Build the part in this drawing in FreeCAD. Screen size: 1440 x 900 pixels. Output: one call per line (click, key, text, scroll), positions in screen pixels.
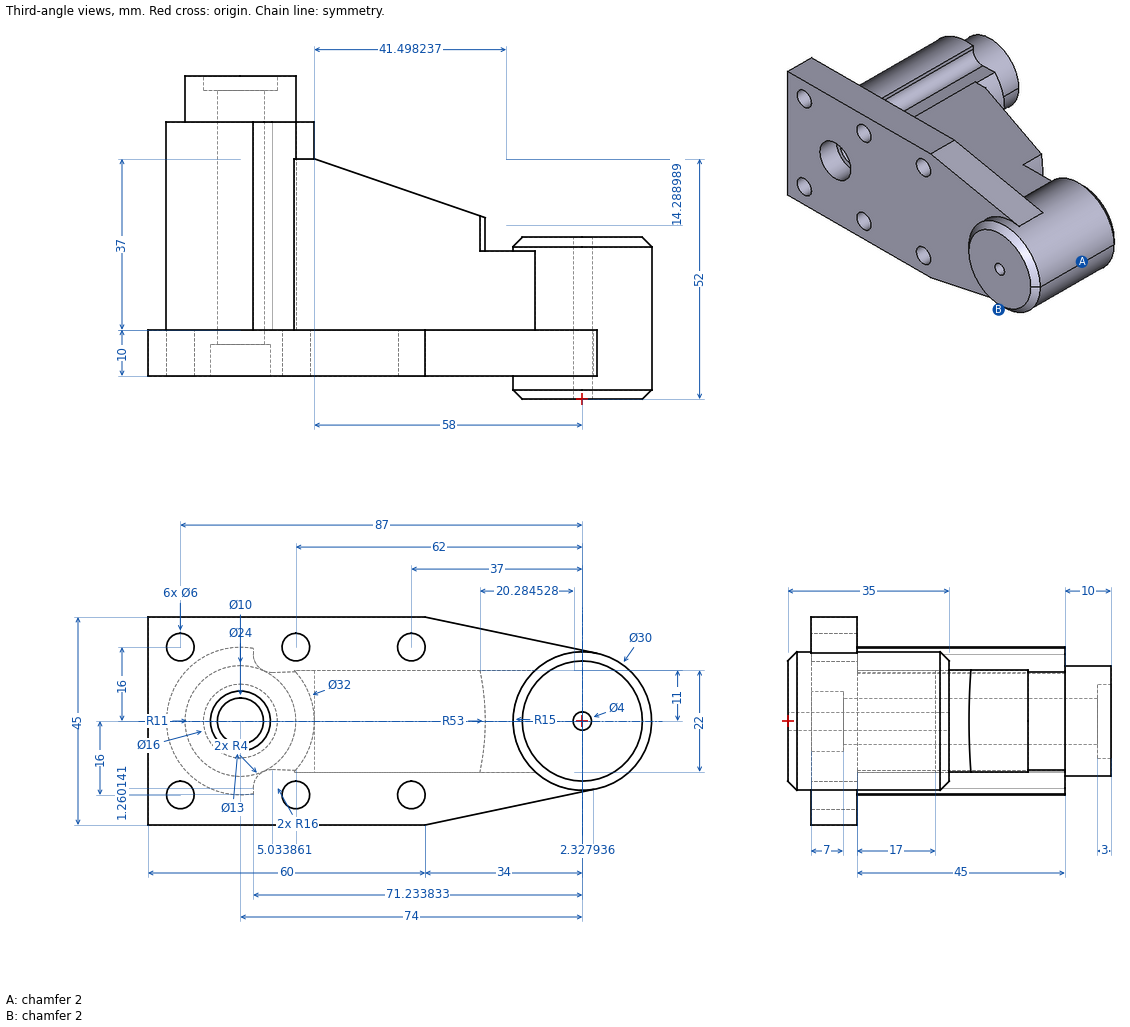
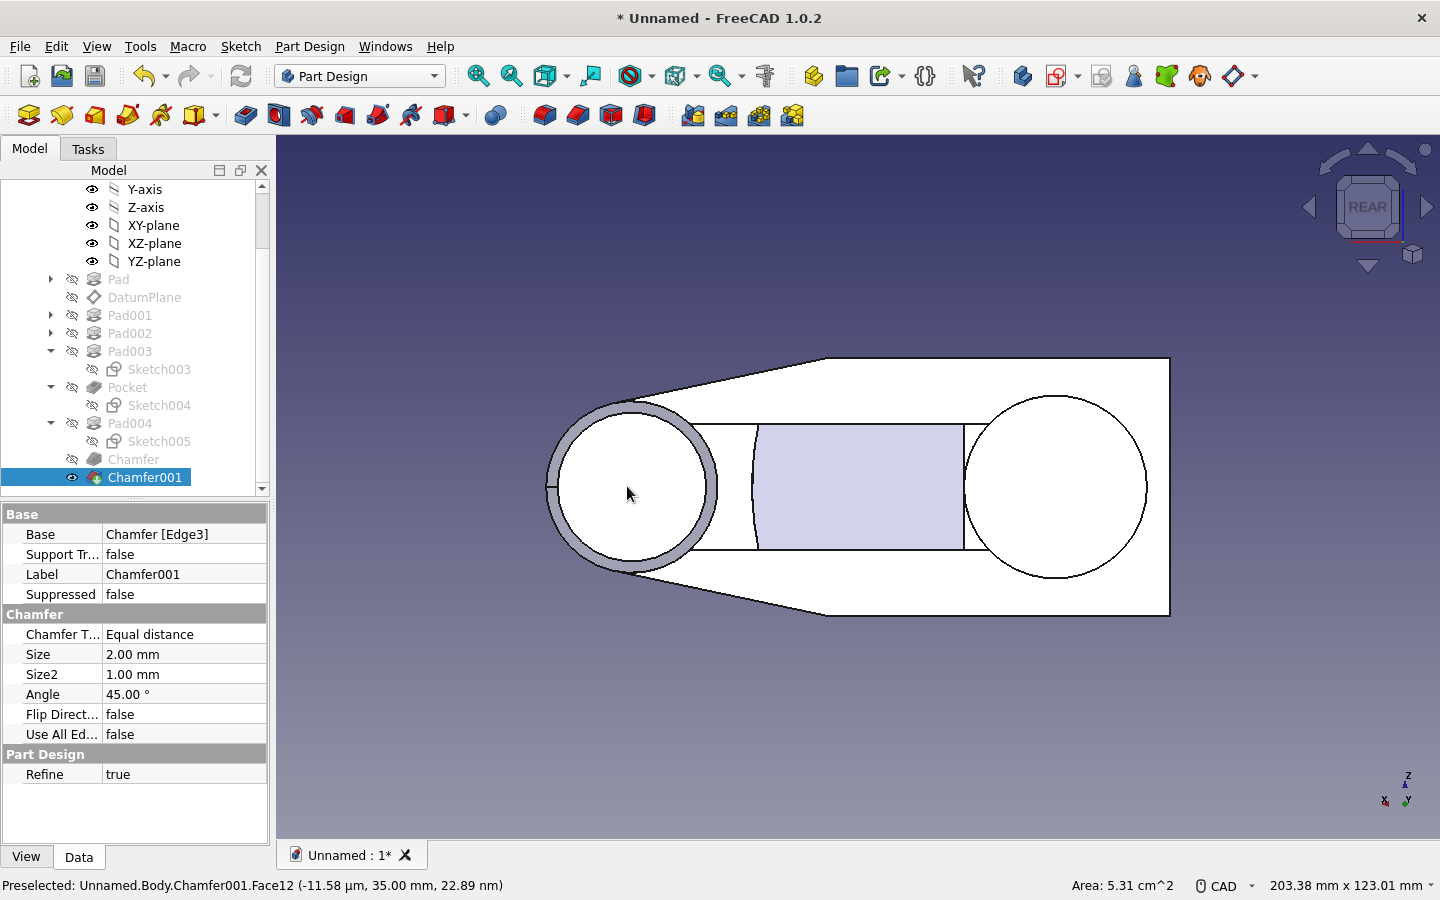
click(1056, 76)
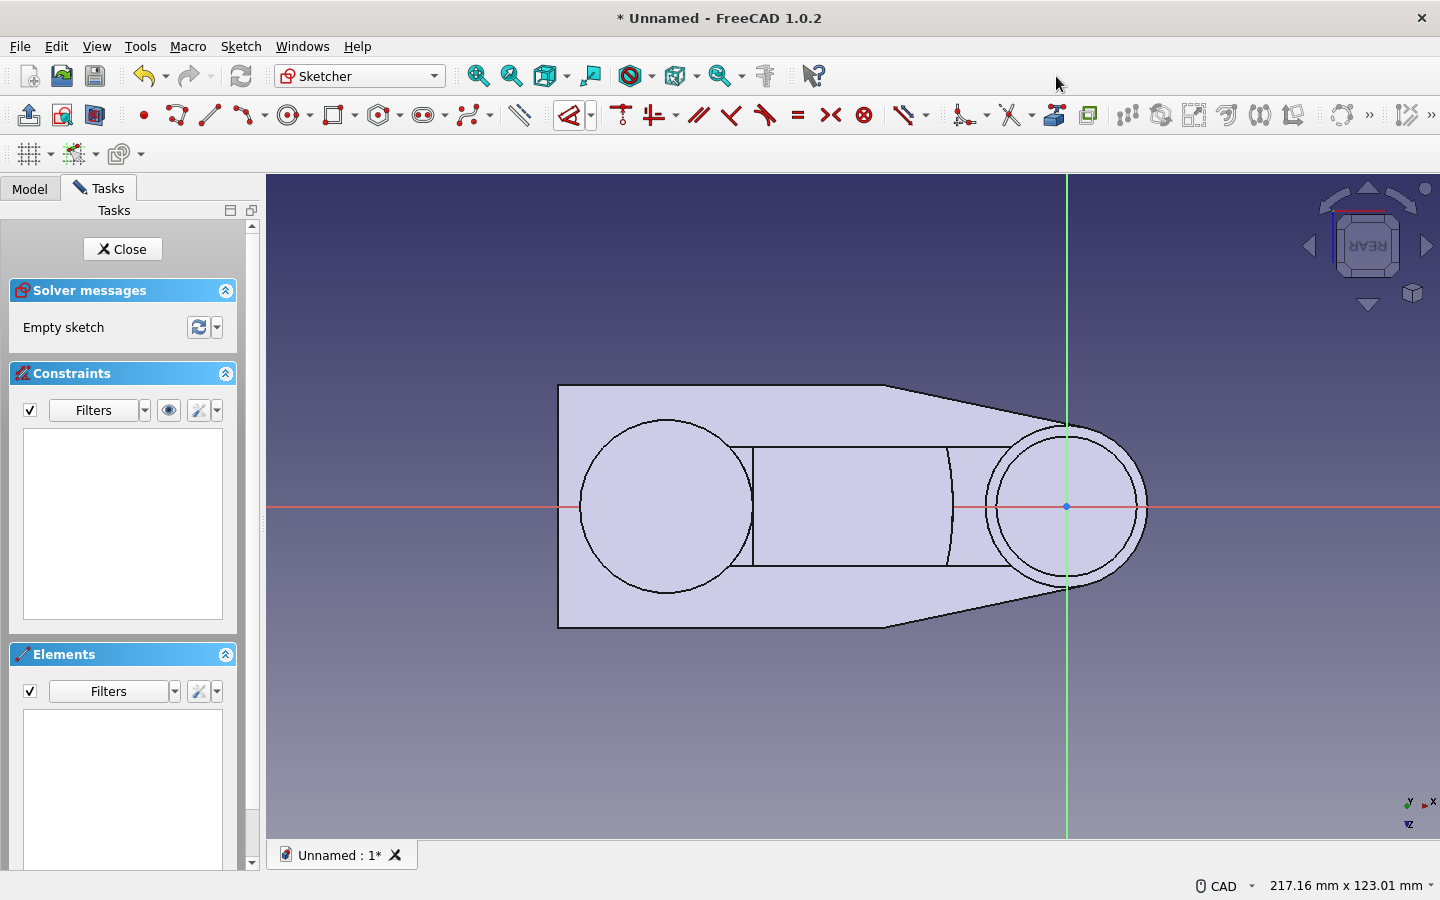
click(95, 116)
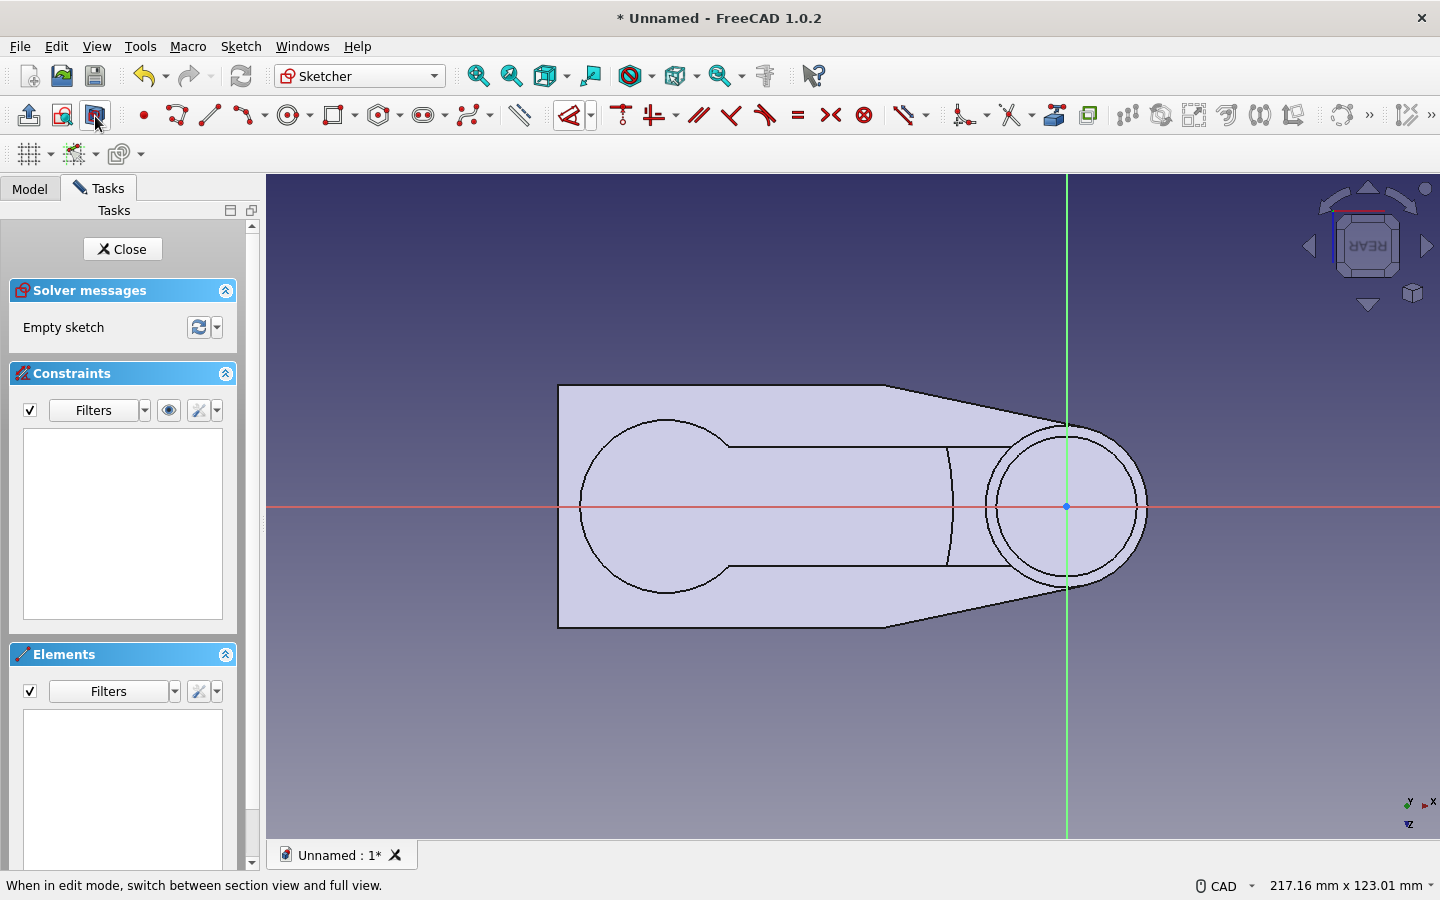
scroll(1081, 506, up, 15)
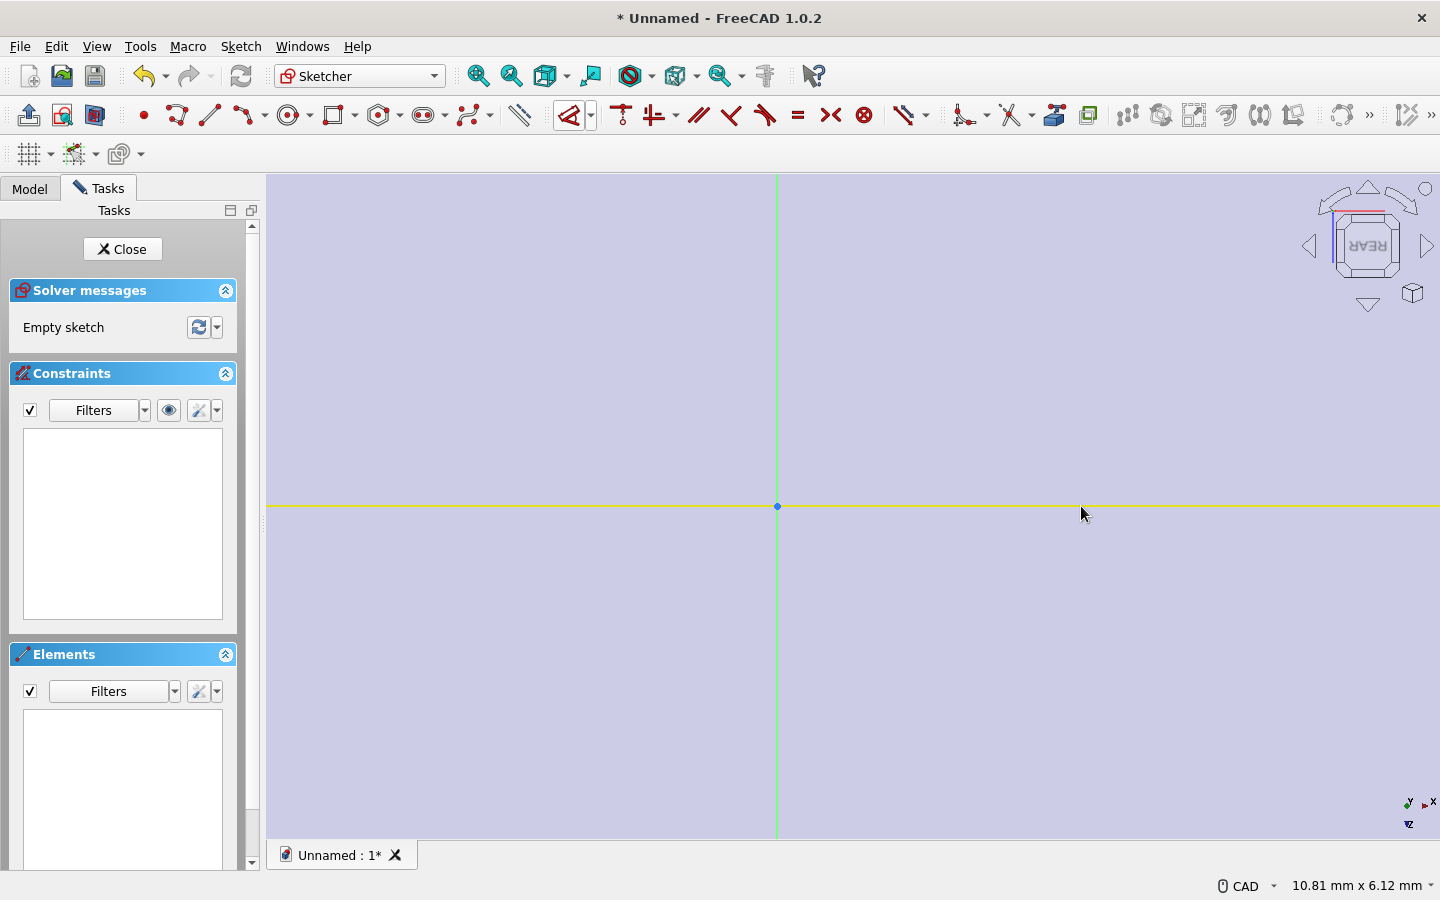
click(288, 116)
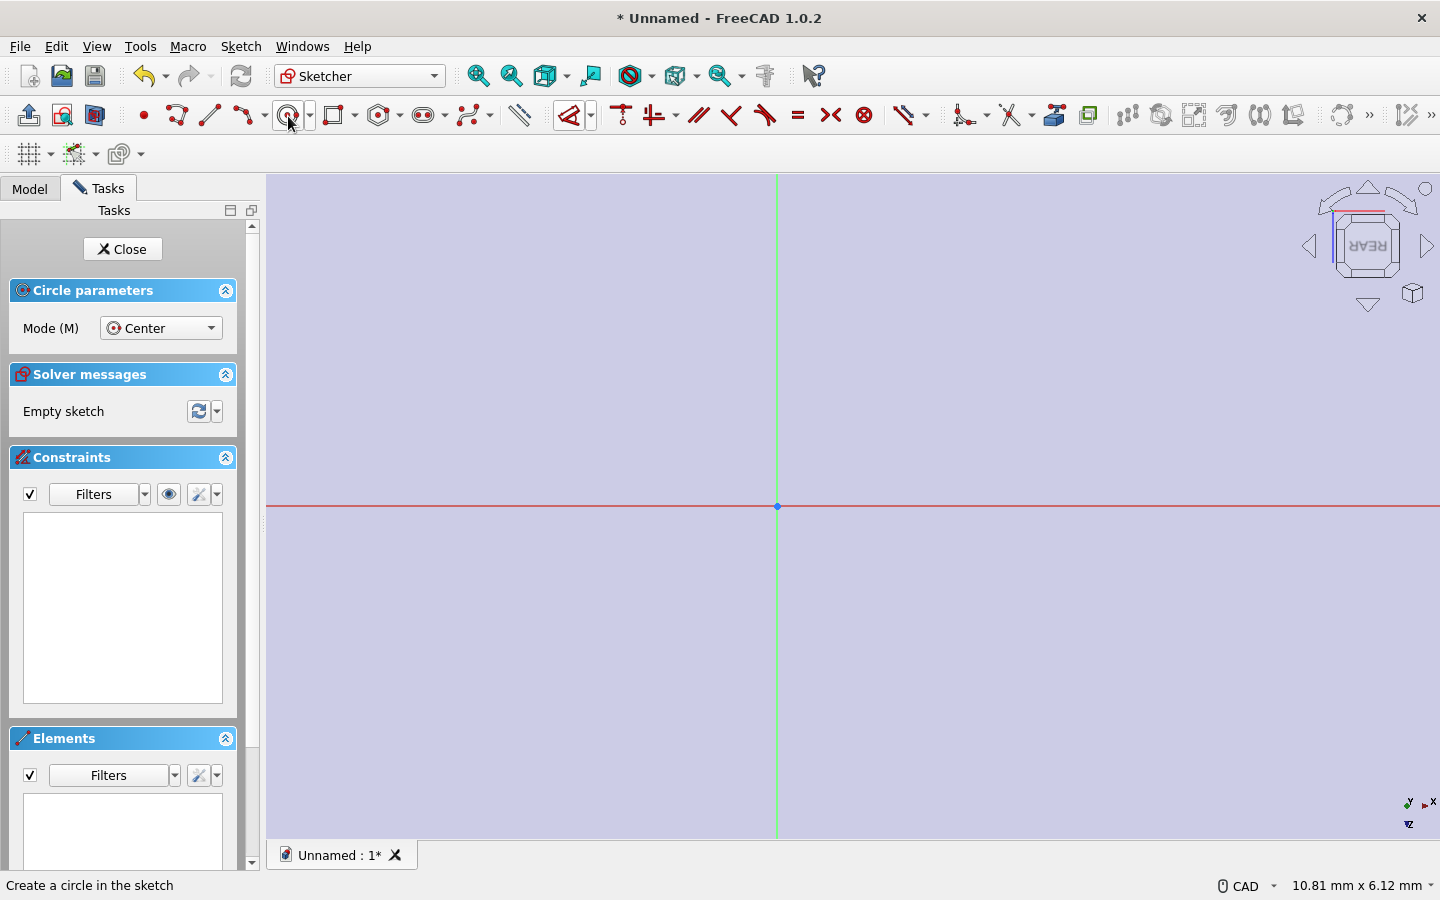
click(777, 506)
click(931, 353)
key(Escape)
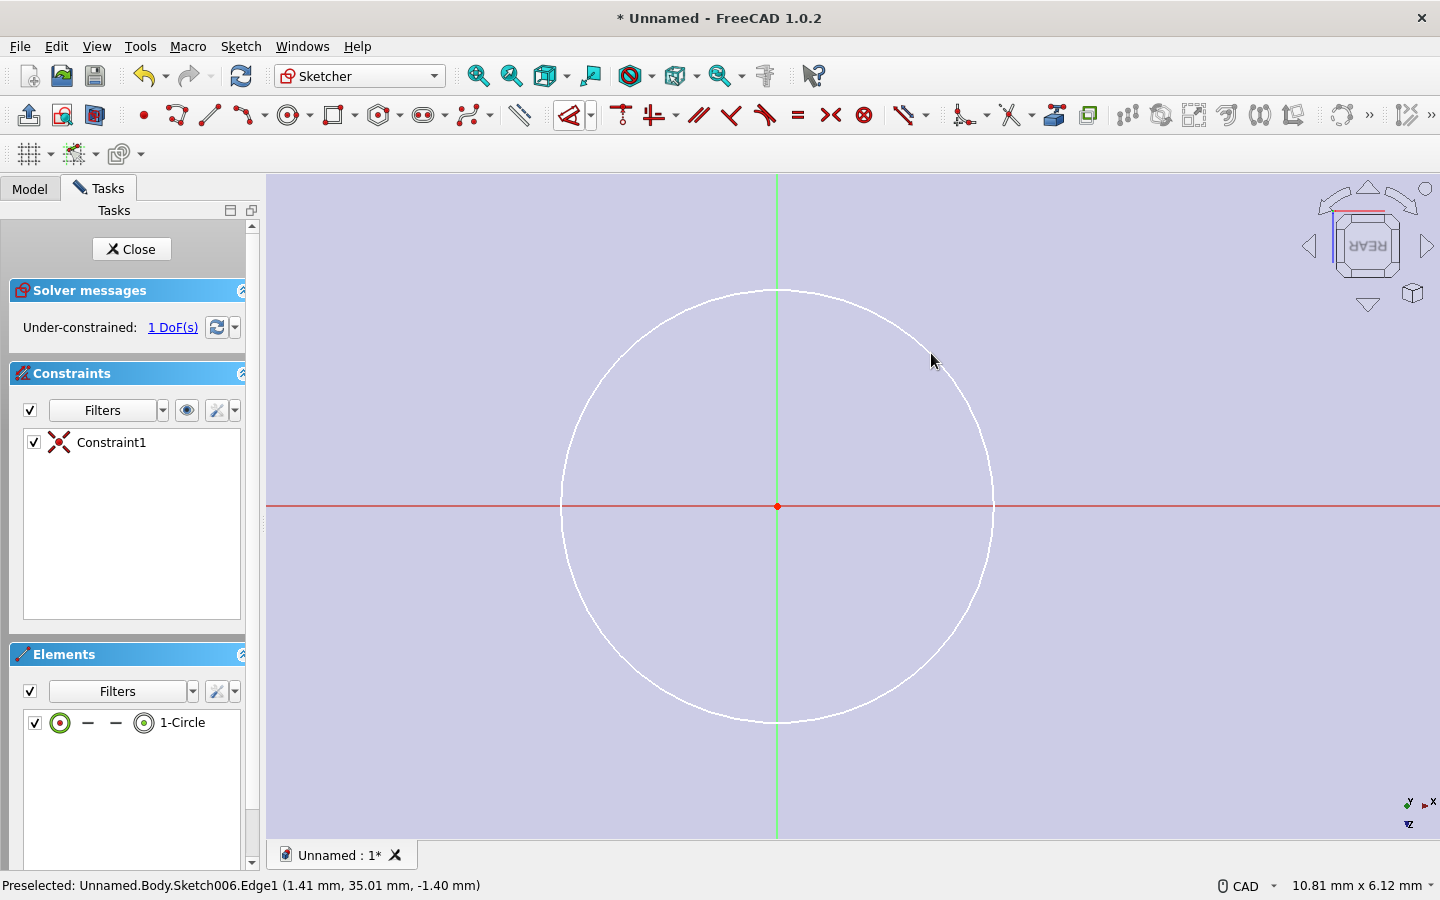
click(930, 353)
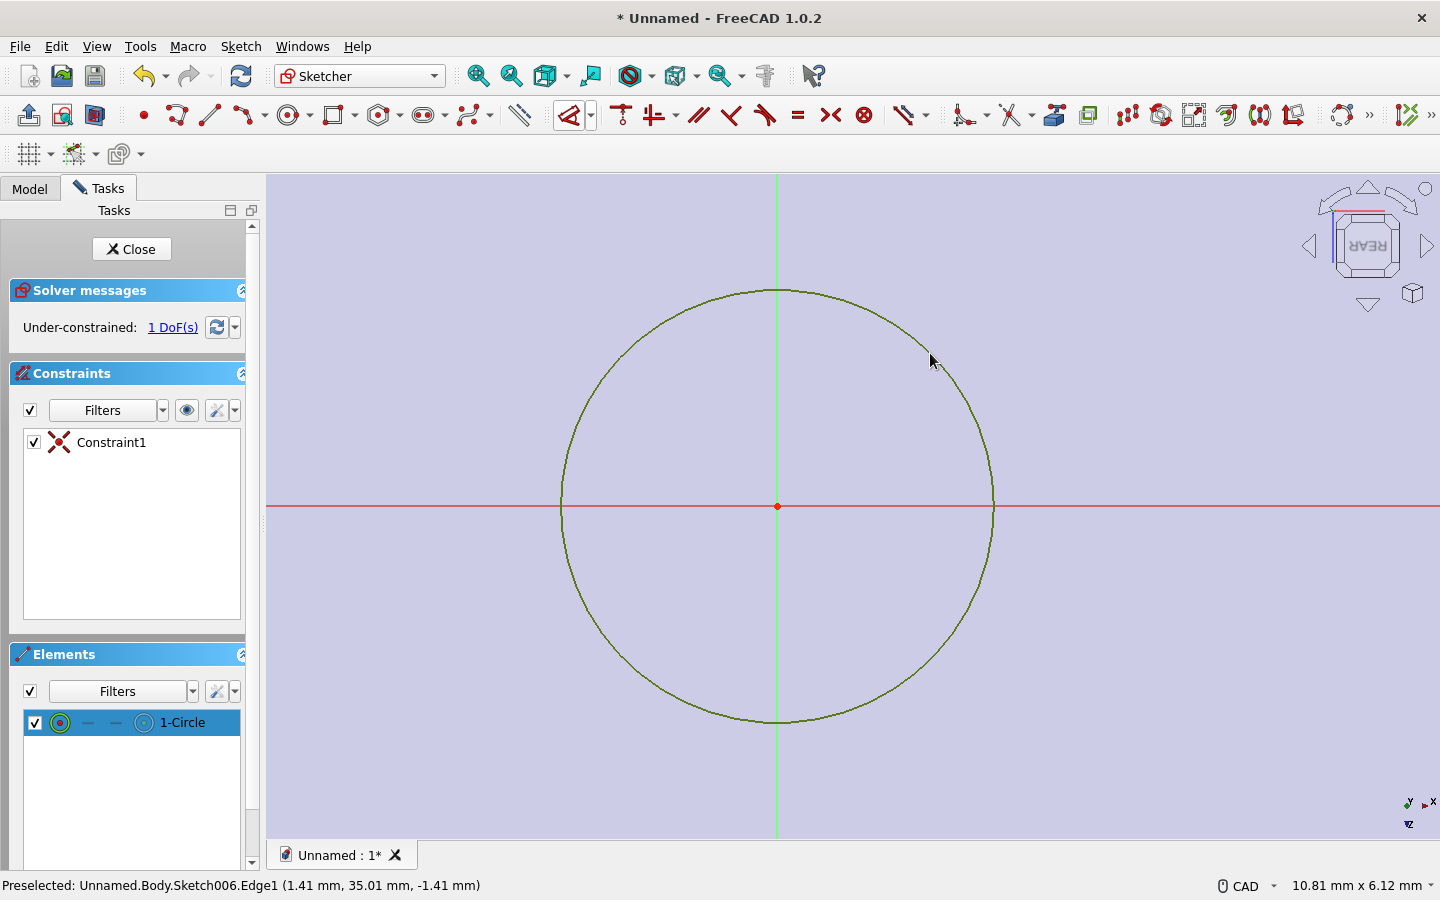
click(590, 116)